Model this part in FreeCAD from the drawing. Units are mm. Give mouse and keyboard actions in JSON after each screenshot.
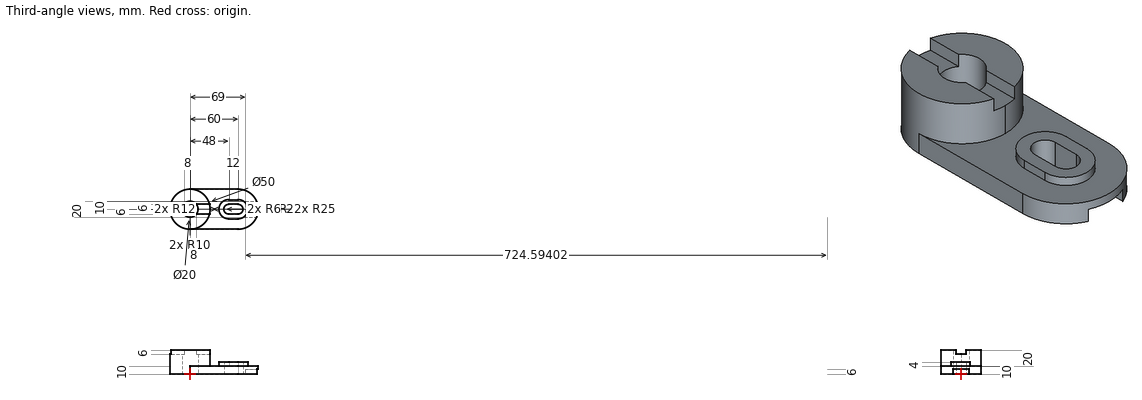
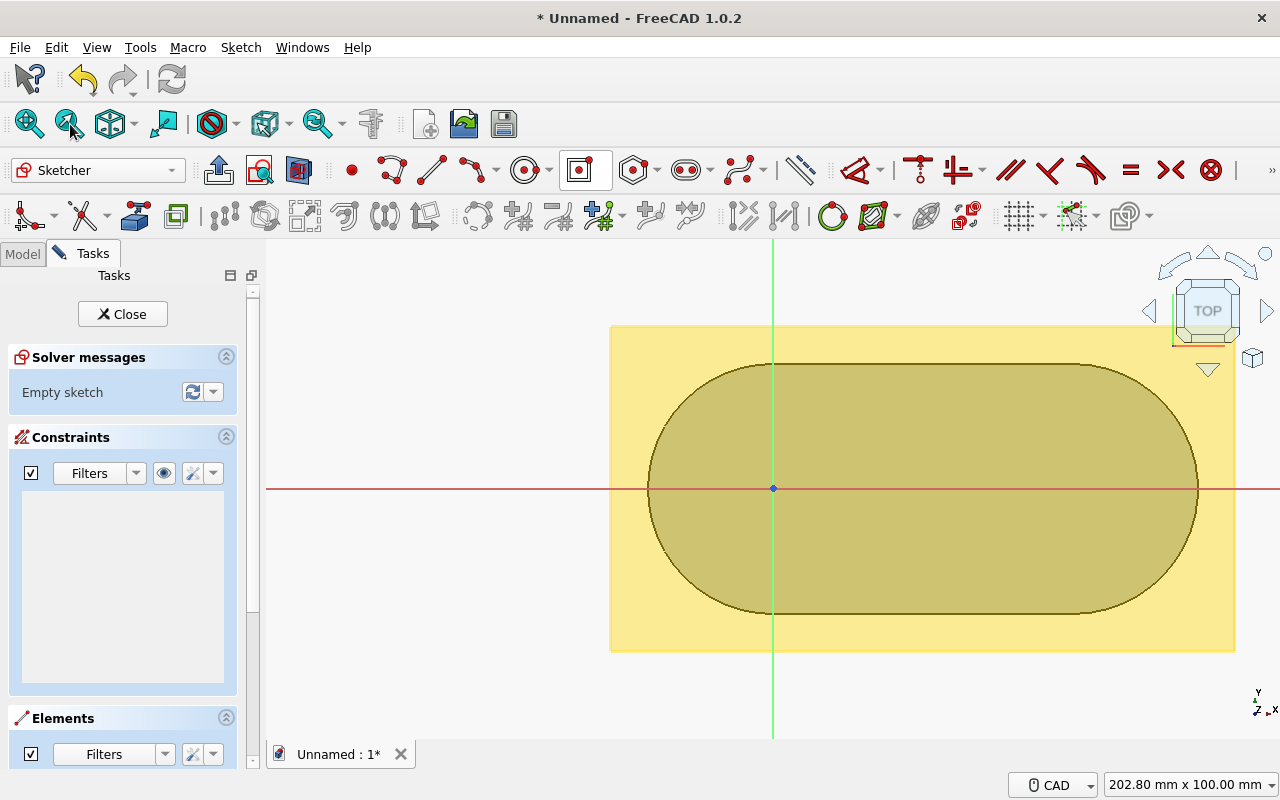
{"action": "left_click", "coordinate": [526, 170]}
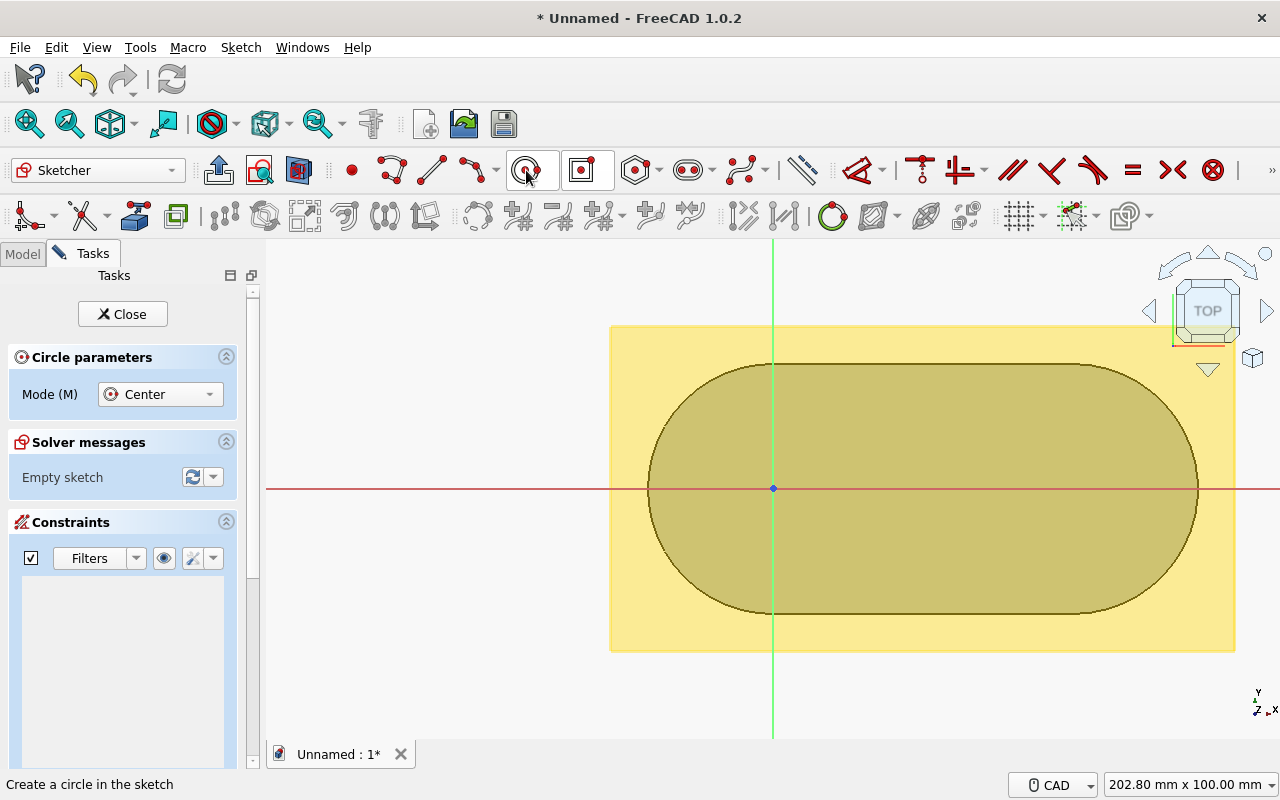
{"action": "left_click", "coordinate": [773, 489]}
{"action": "left_click", "coordinate": [861, 401]}
{"action": "key", "text": "Escape"}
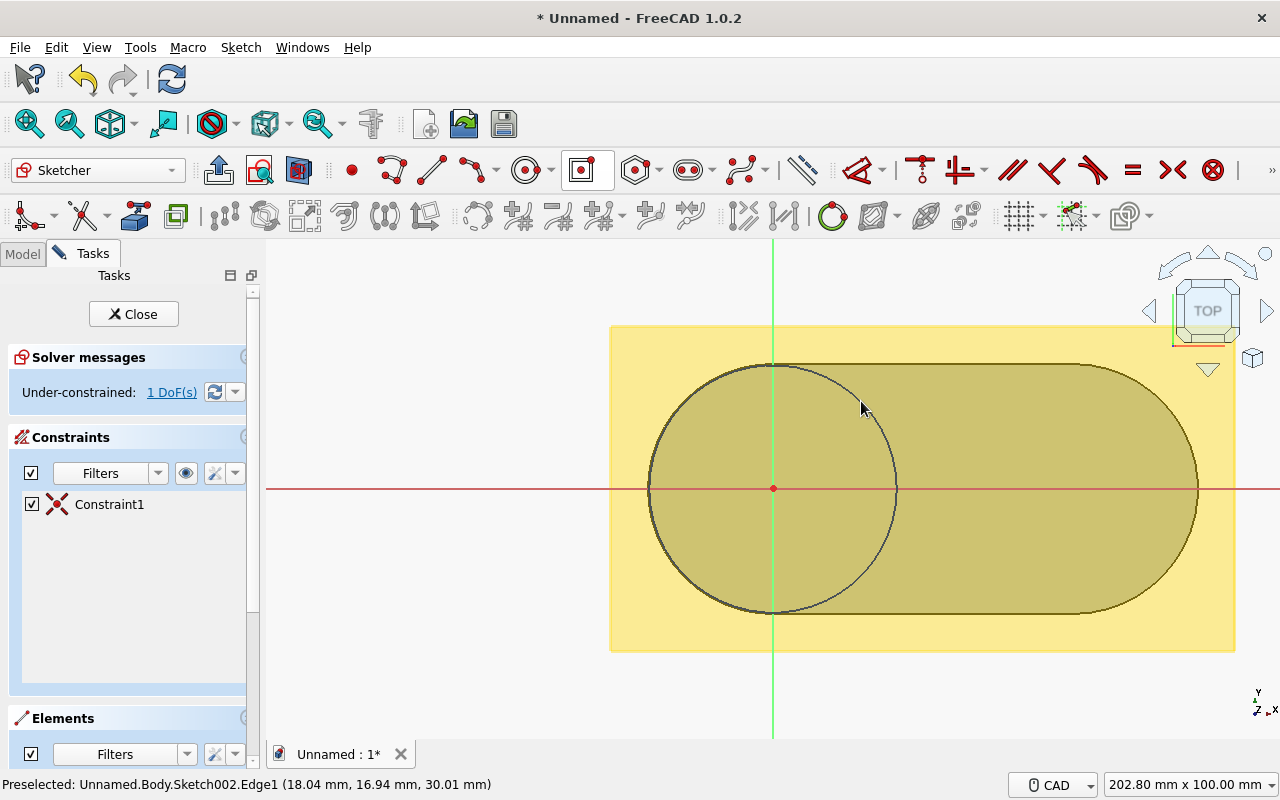
{"action": "left_click", "coordinate": [858, 170]}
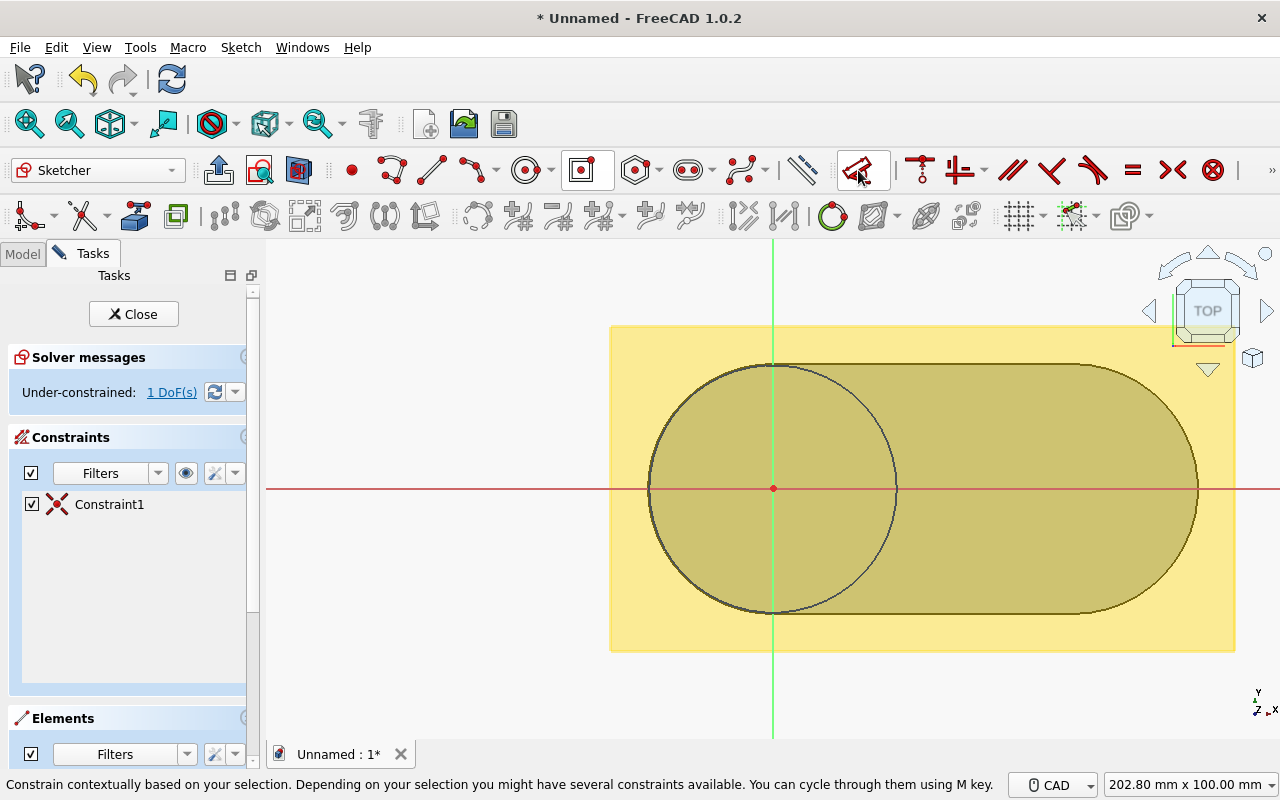
{"action": "left_click", "coordinate": [860, 401]}
{"action": "left_click", "coordinate": [882, 378]}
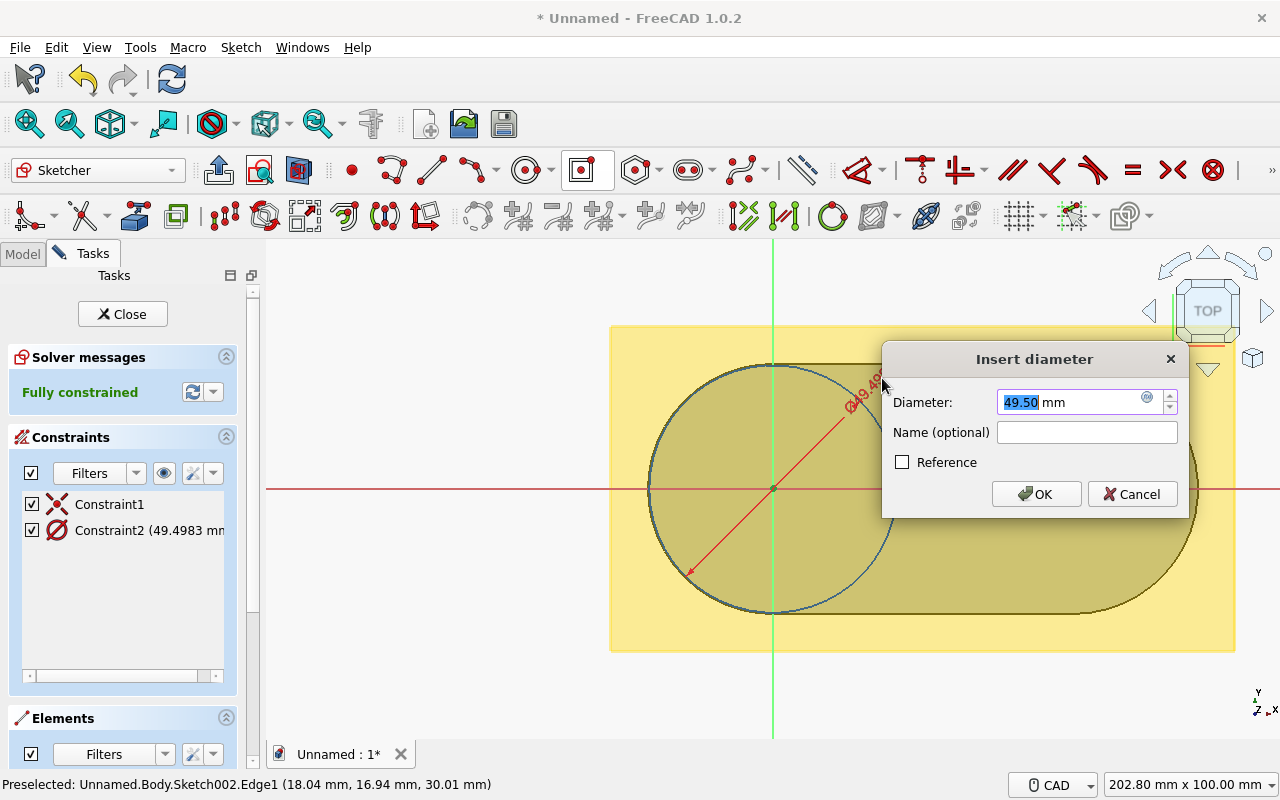
{"action": "type", "text": "50"}
{"action": "key", "text": "Return"}
{"action": "key", "text": "Escape"}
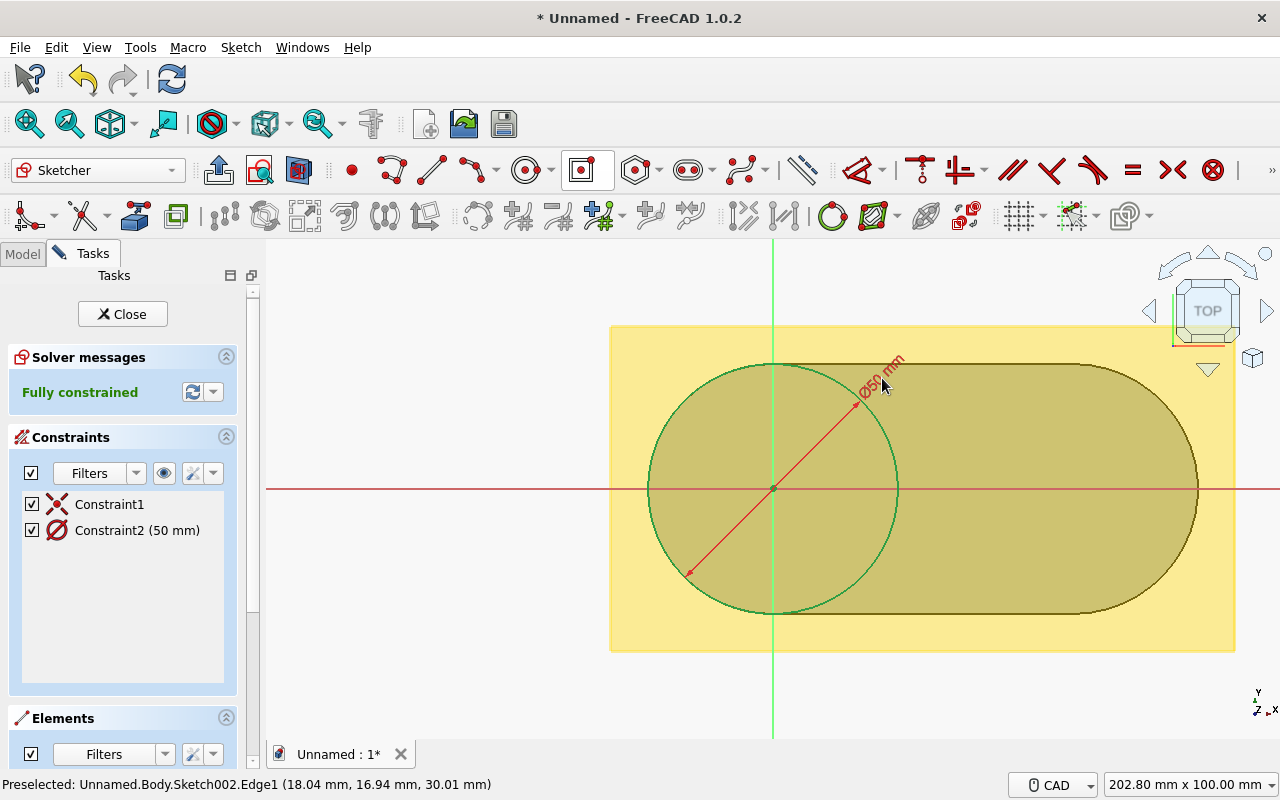
{"action": "left_click", "coordinate": [123, 314]}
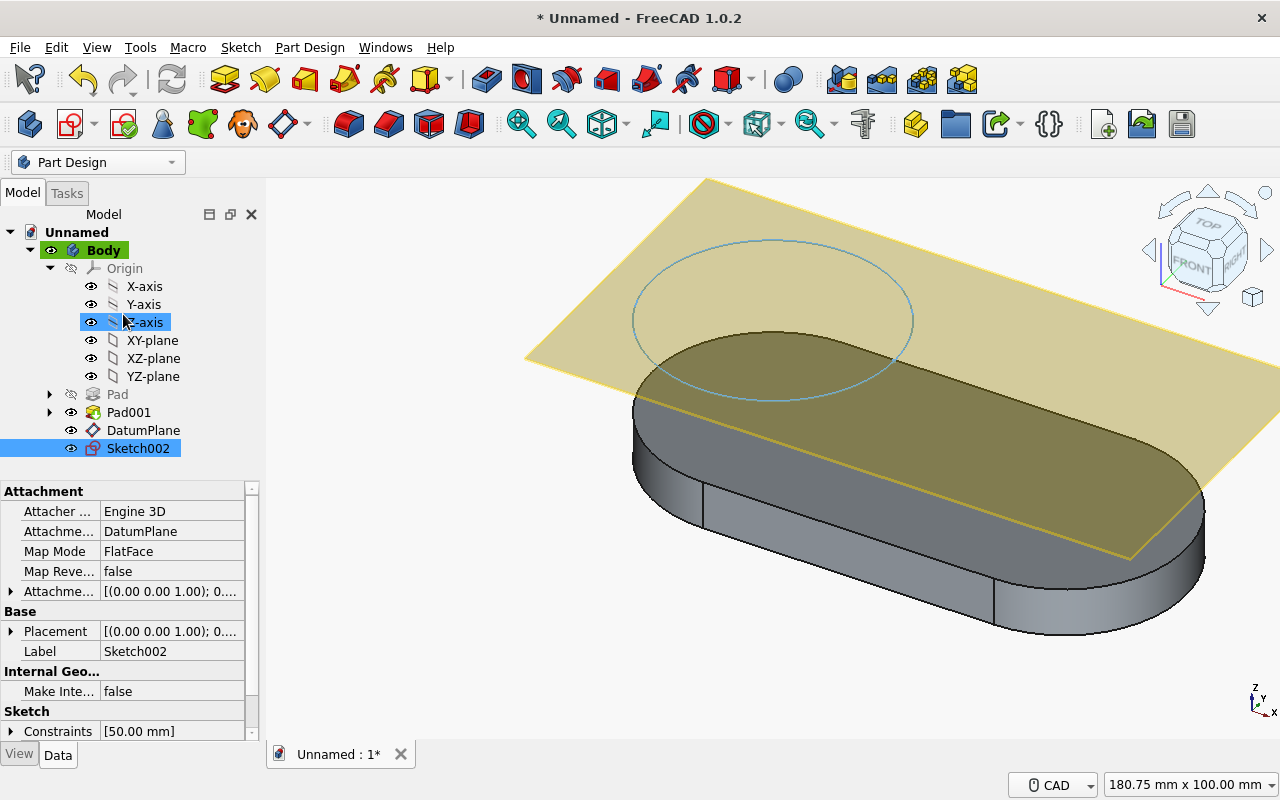
{"action": "left_click", "coordinate": [226, 80]}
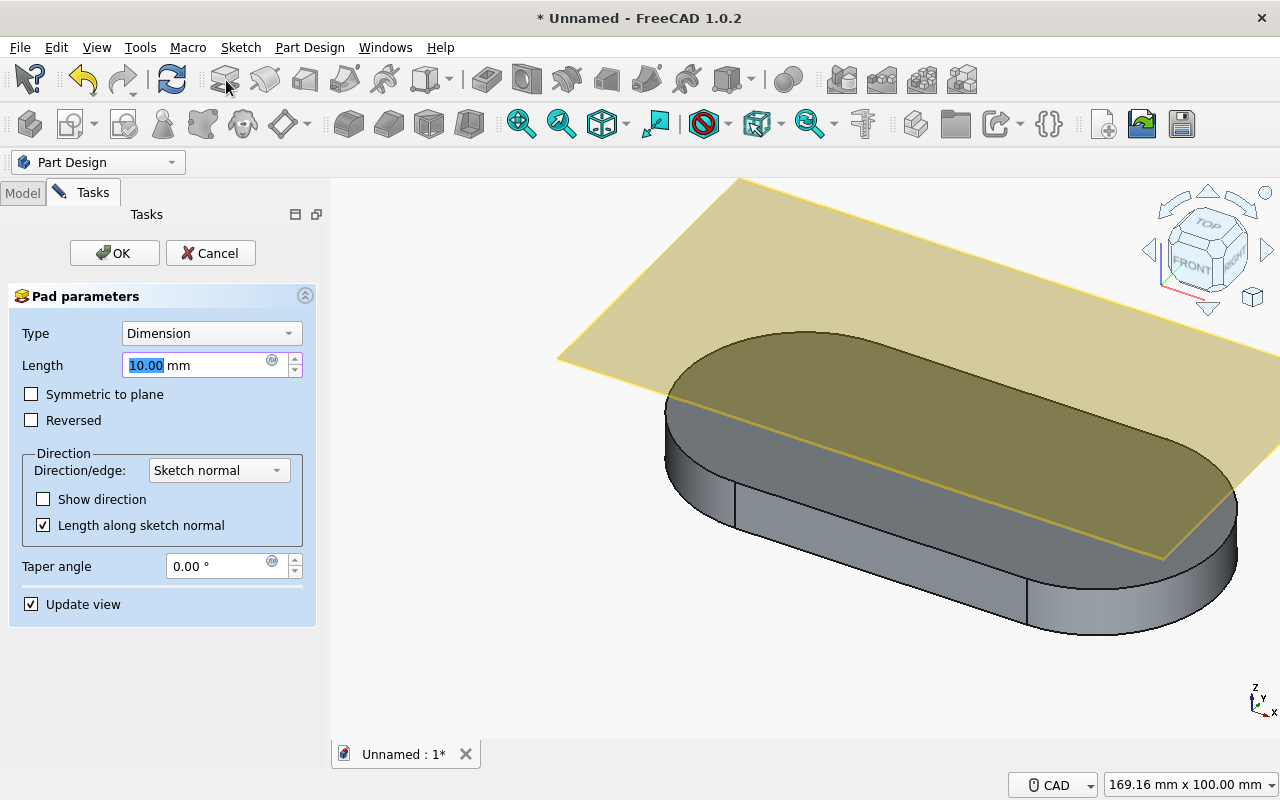
{"action": "type", "text": "20"}
{"action": "key", "text": "Tab"}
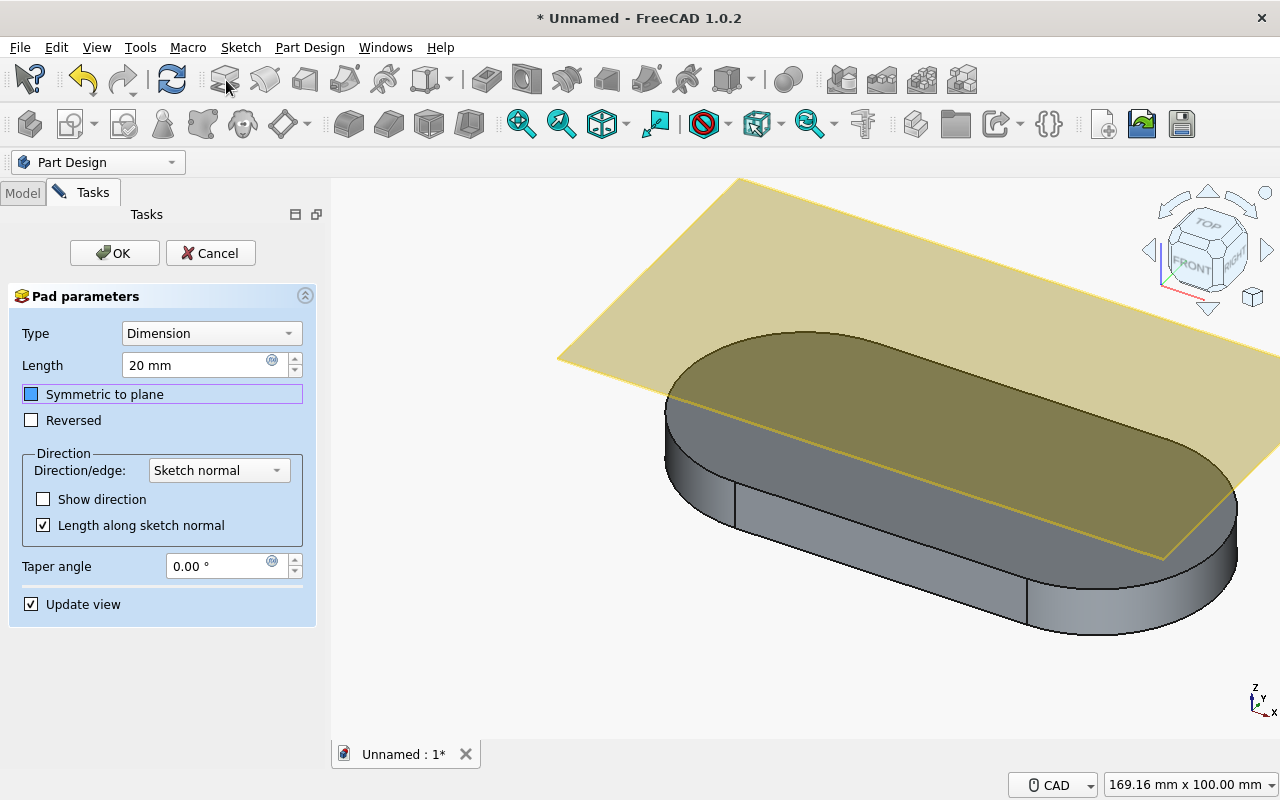
{"action": "left_click", "coordinate": [30, 420]}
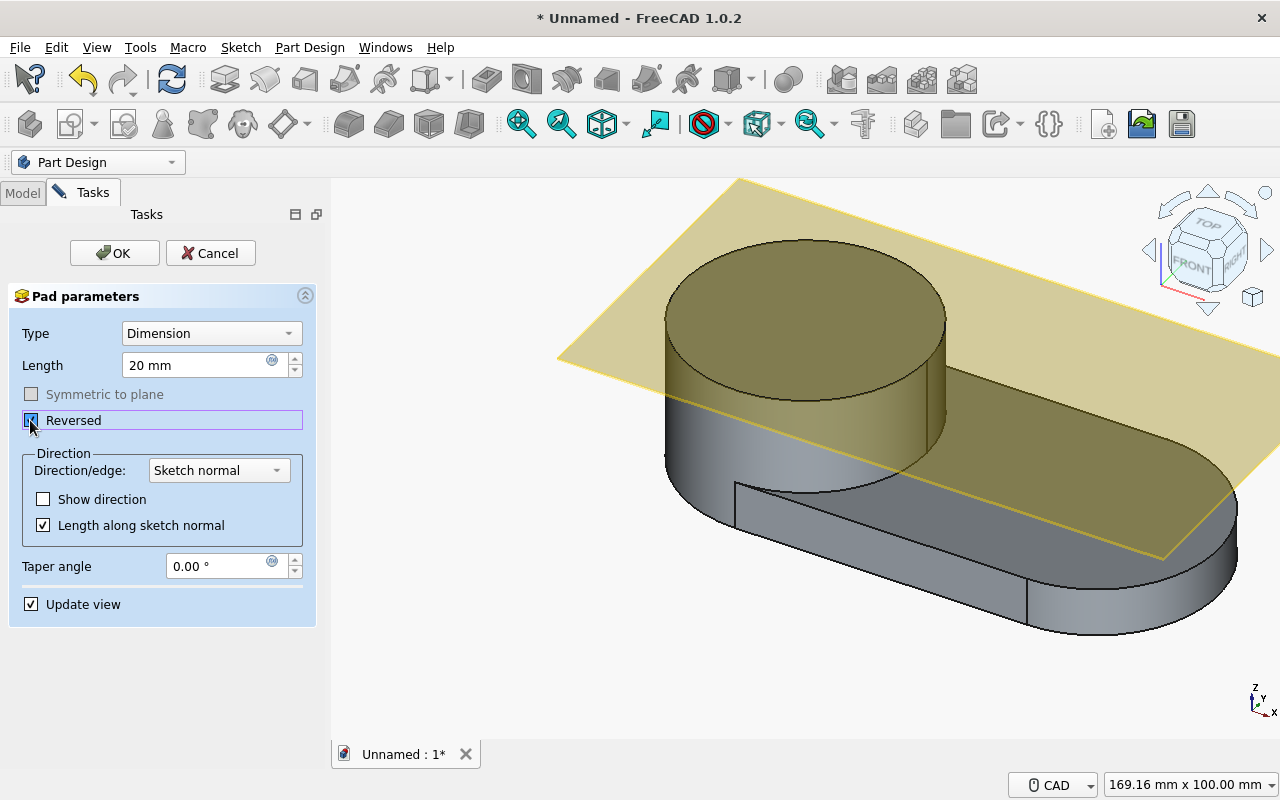
{"action": "left_click", "coordinate": [115, 253]}